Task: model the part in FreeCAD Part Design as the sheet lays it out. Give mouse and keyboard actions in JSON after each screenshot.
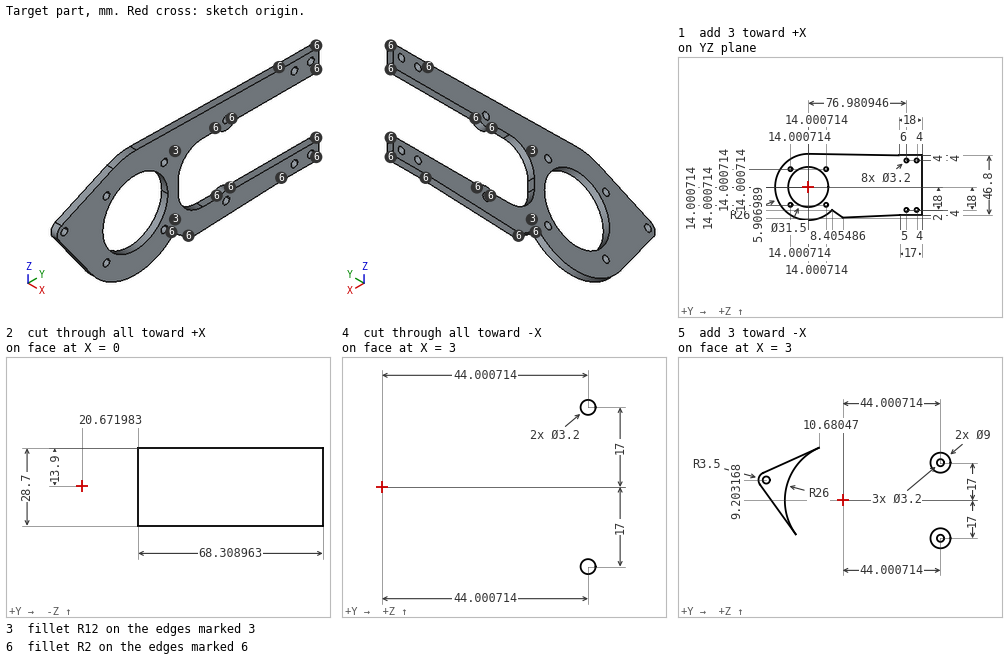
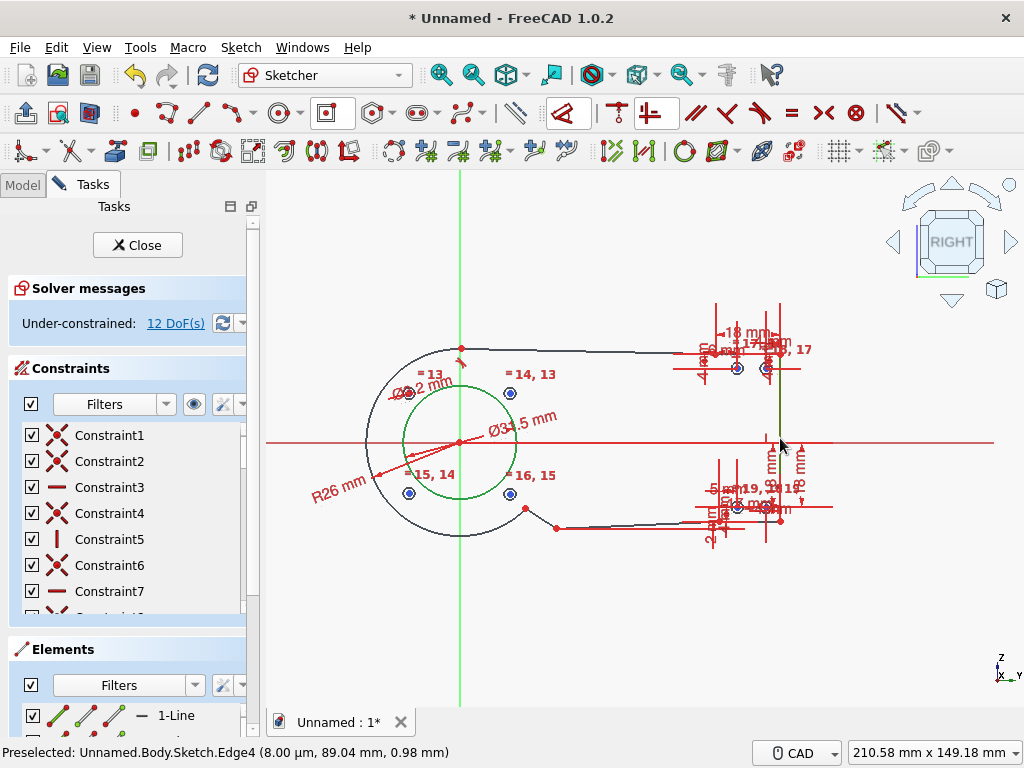
{"action": "left_click", "coordinate": [586, 114]}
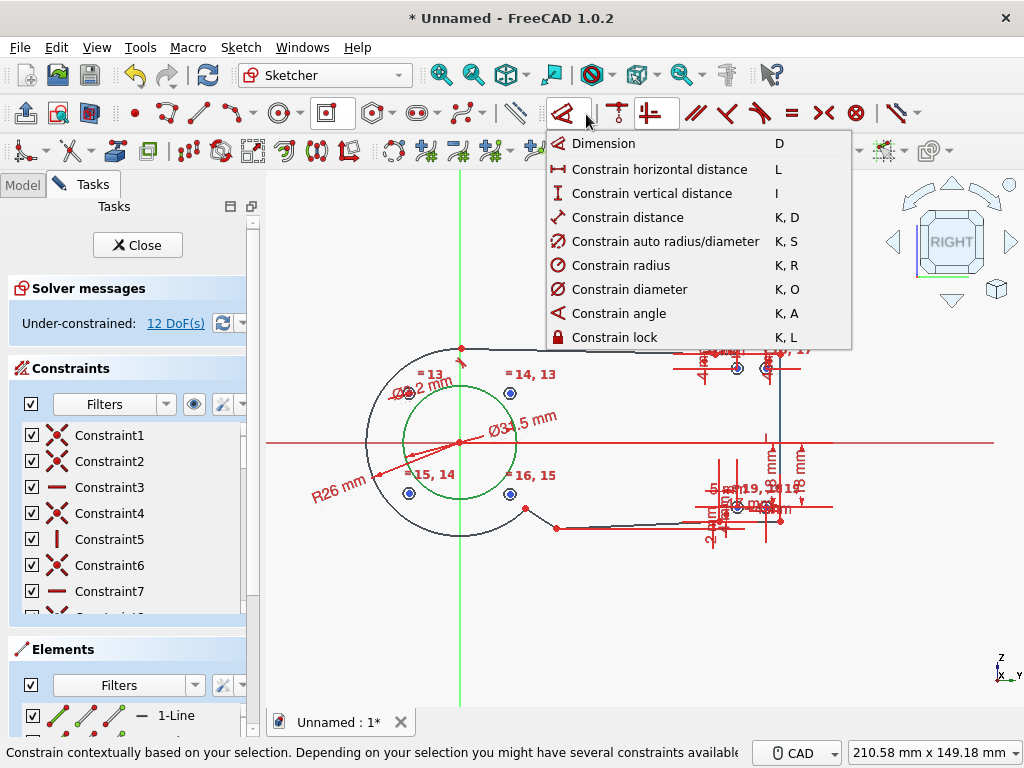
{"action": "left_click", "coordinate": [699, 193]}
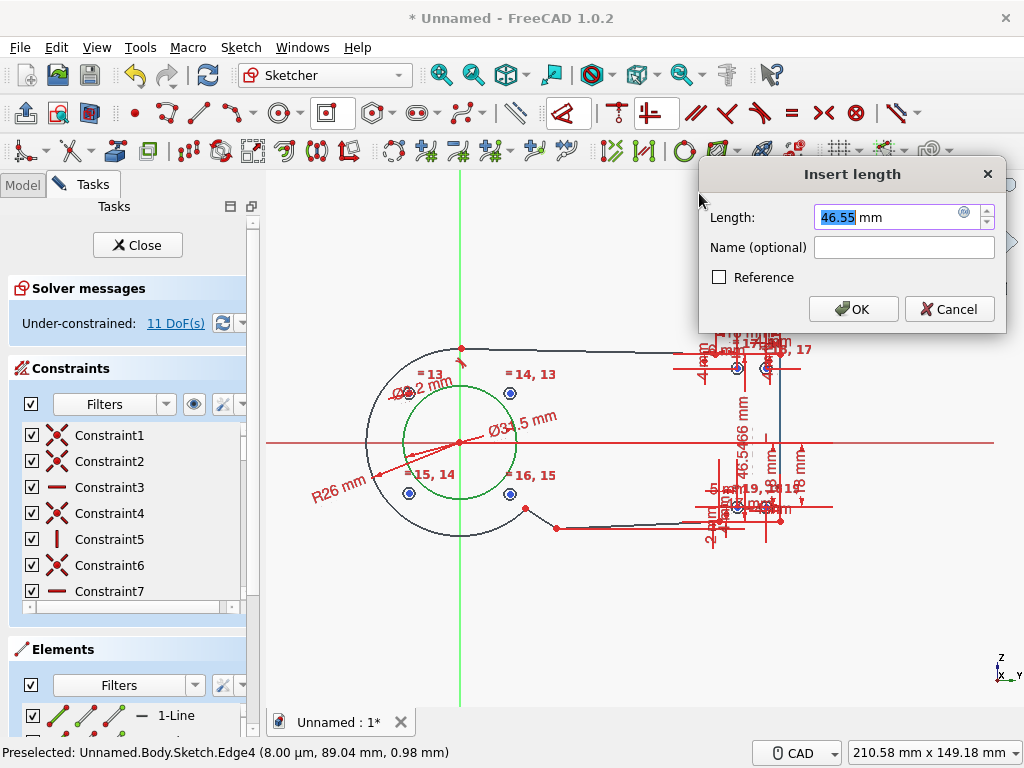
{"action": "type", "text": "46.8"}
{"action": "key", "text": "Return"}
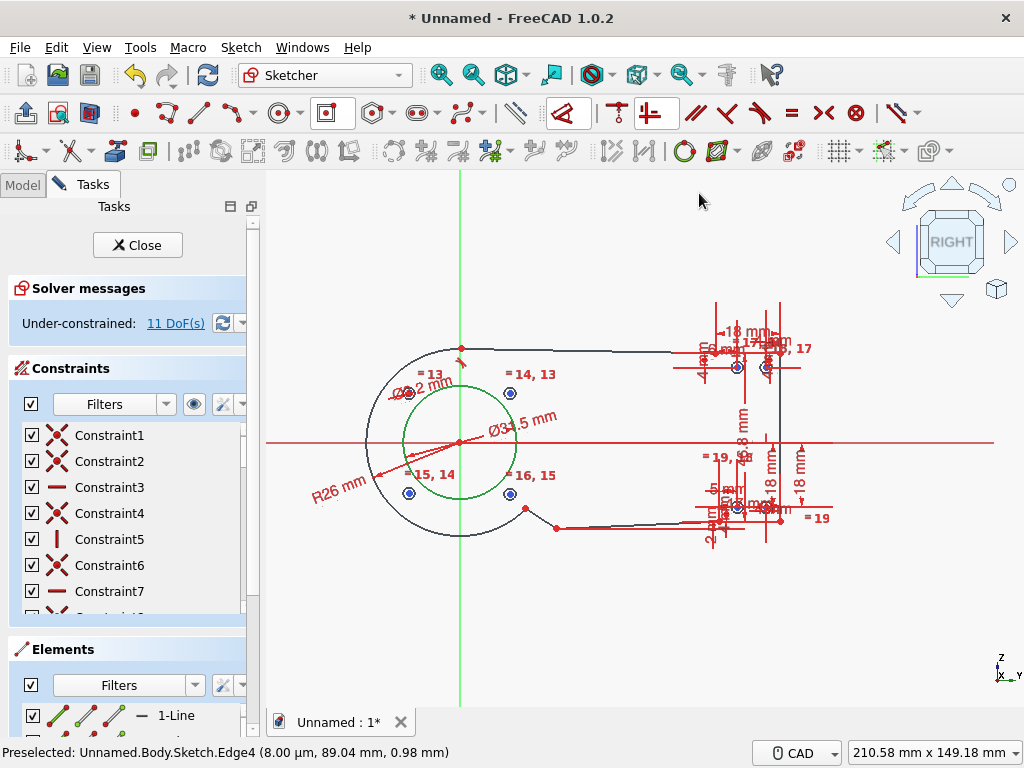
{"action": "scroll", "coordinate": [535, 515], "scroll_direction": "up", "scroll_amount": 2}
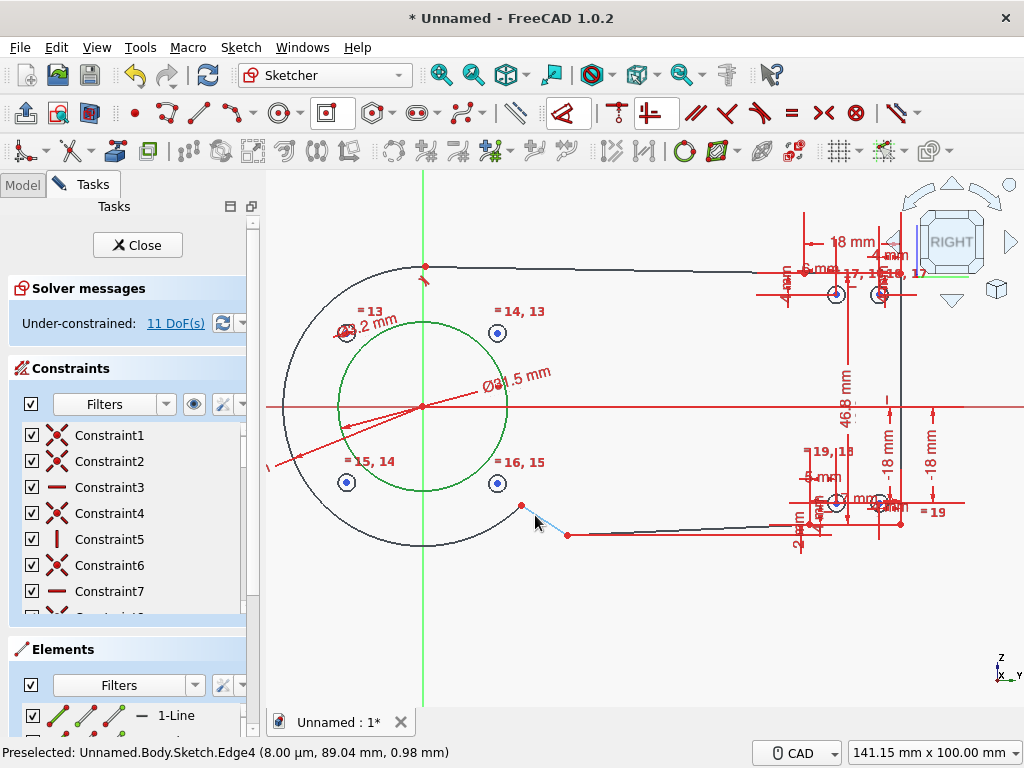
{"action": "left_click", "coordinate": [535, 514]}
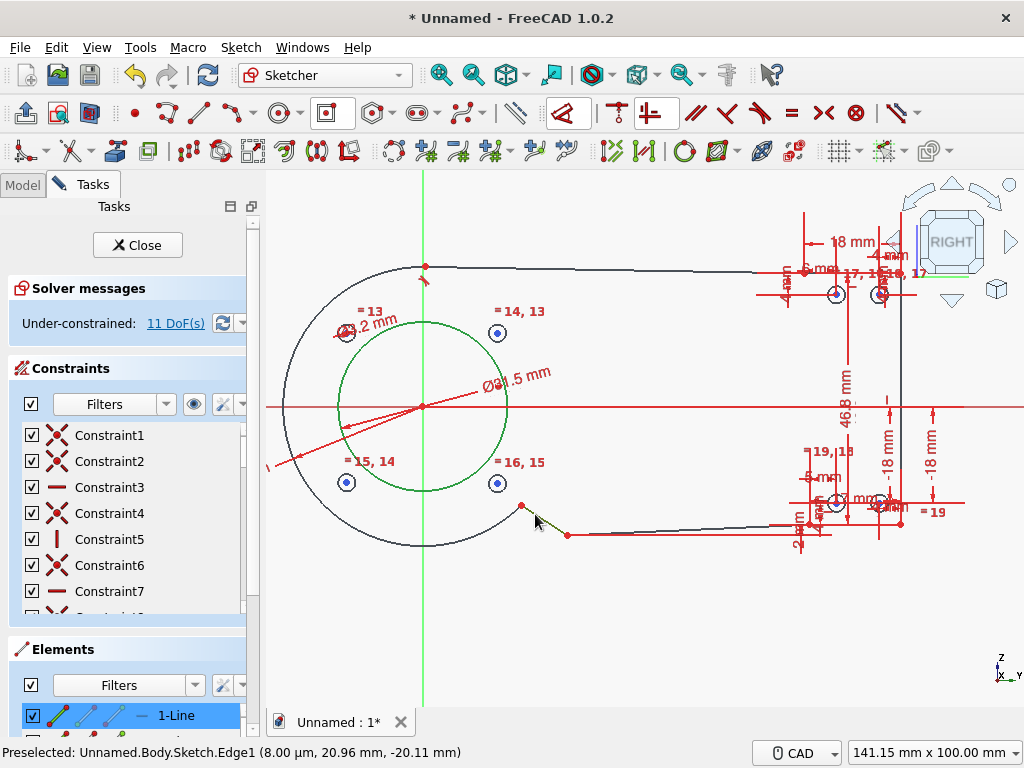
{"action": "left_click", "coordinate": [586, 114]}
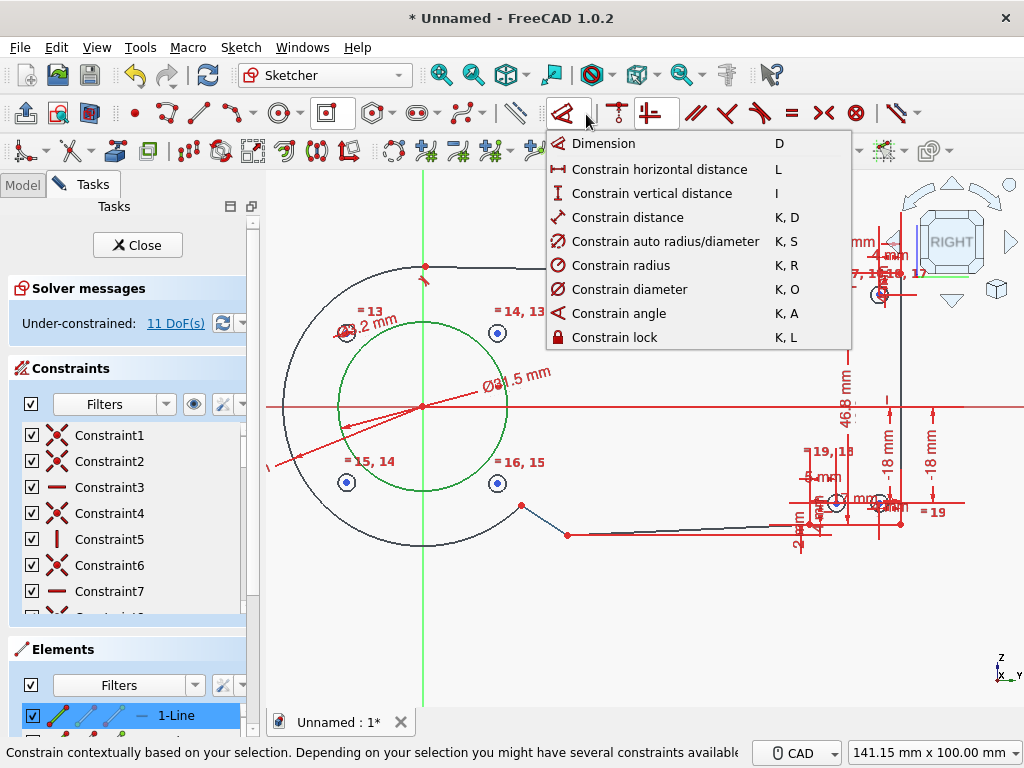
{"action": "left_click", "coordinate": [699, 169]}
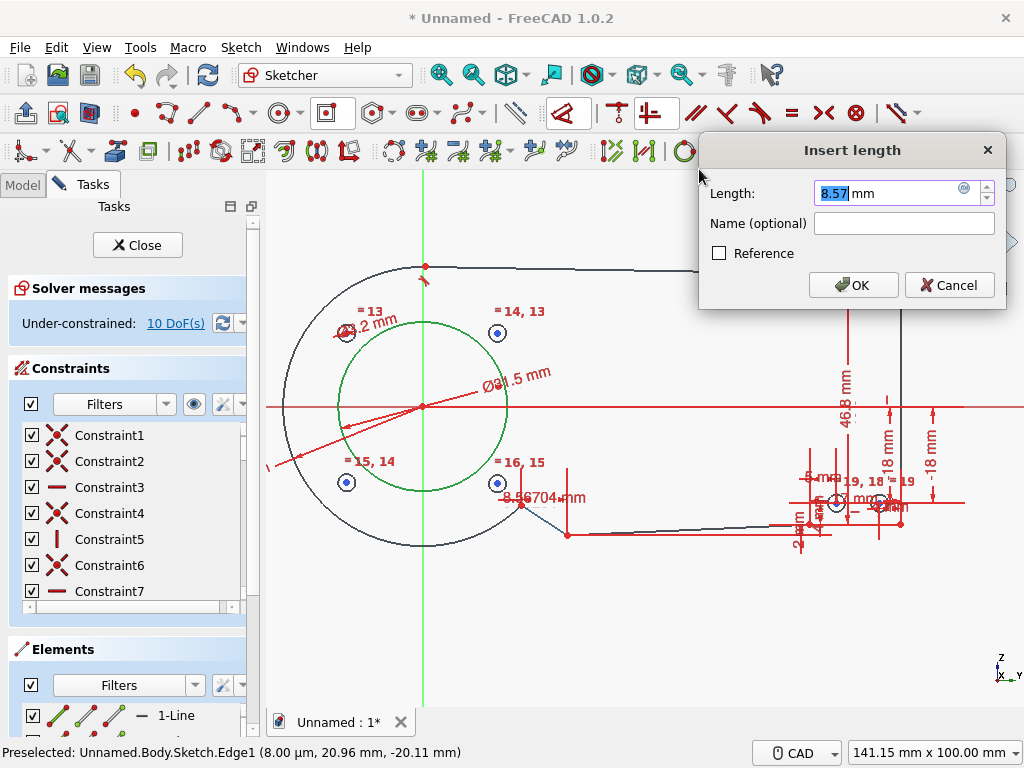
{"action": "type", "text": "8.405486"}
{"action": "key", "text": "Return"}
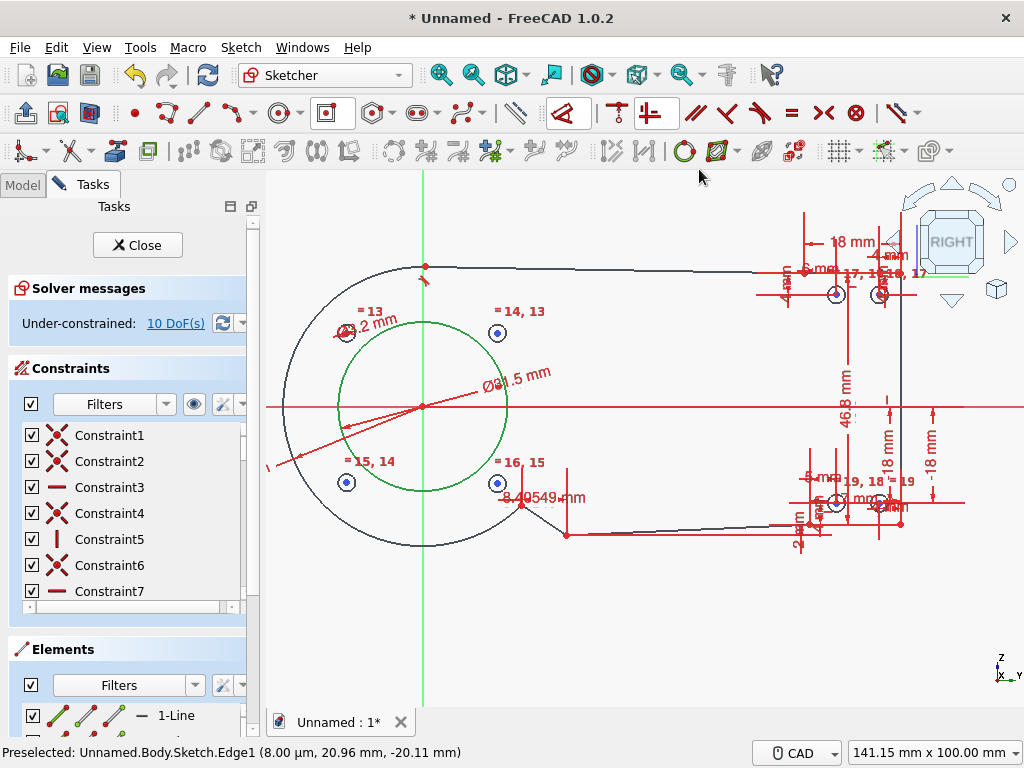
{"action": "scroll", "coordinate": [535, 514], "scroll_direction": "up", "scroll_amount": 2}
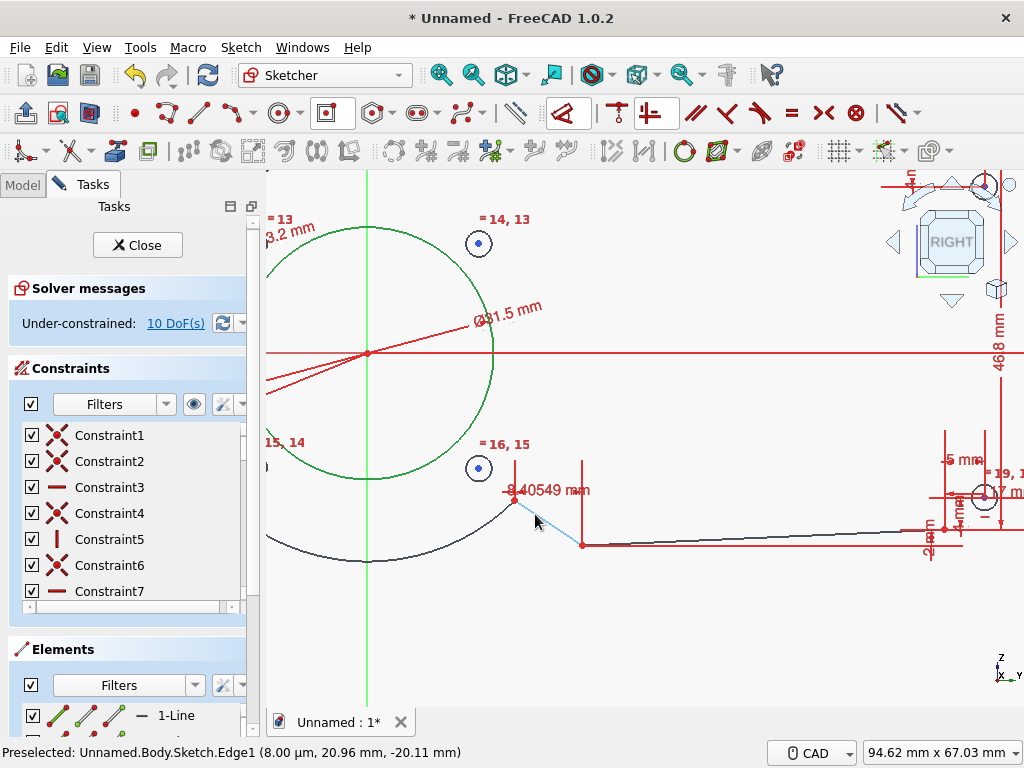
{"action": "left_click", "coordinate": [535, 514]}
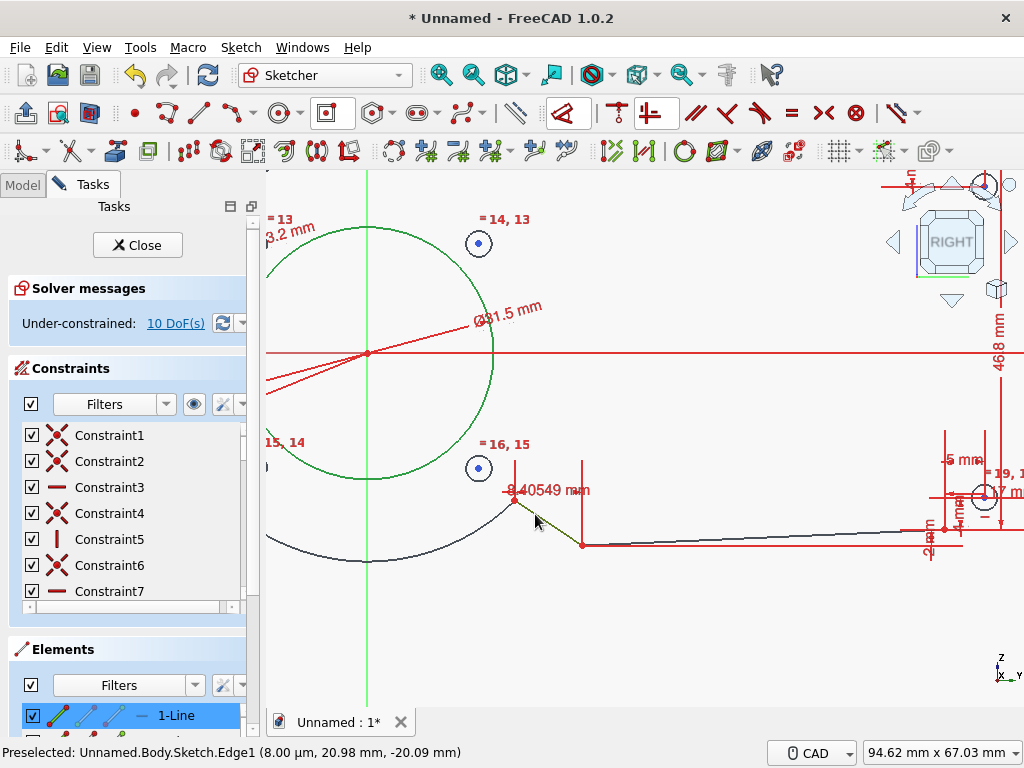
{"action": "left_click", "coordinate": [586, 114]}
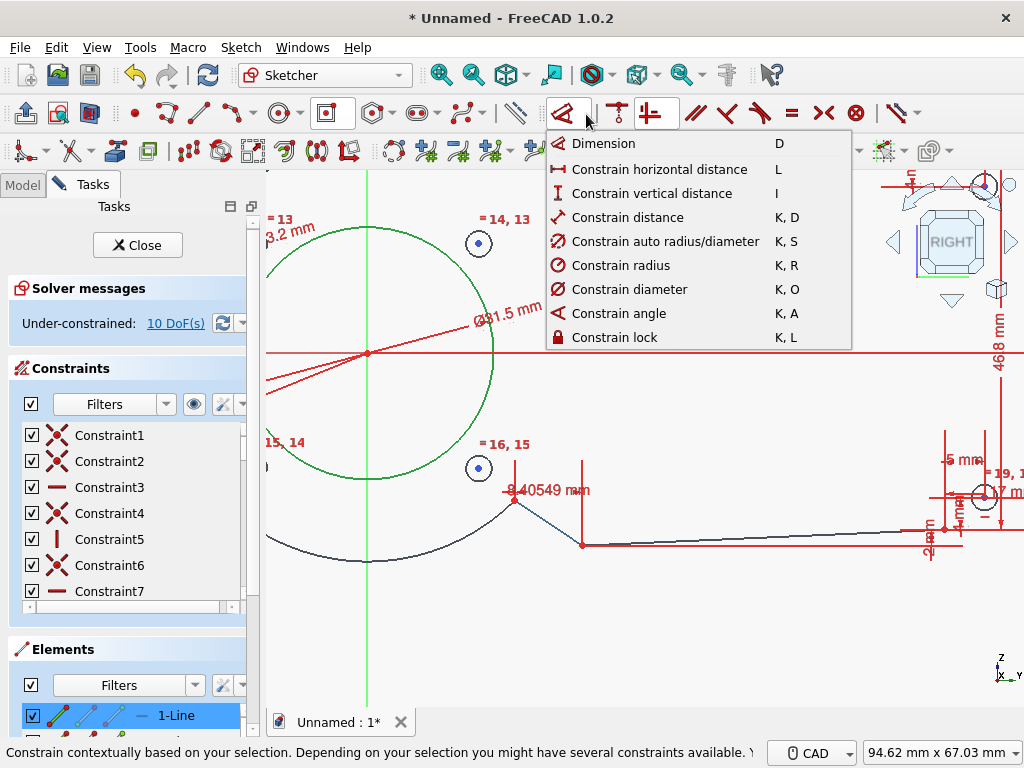
{"action": "left_click", "coordinate": [699, 193]}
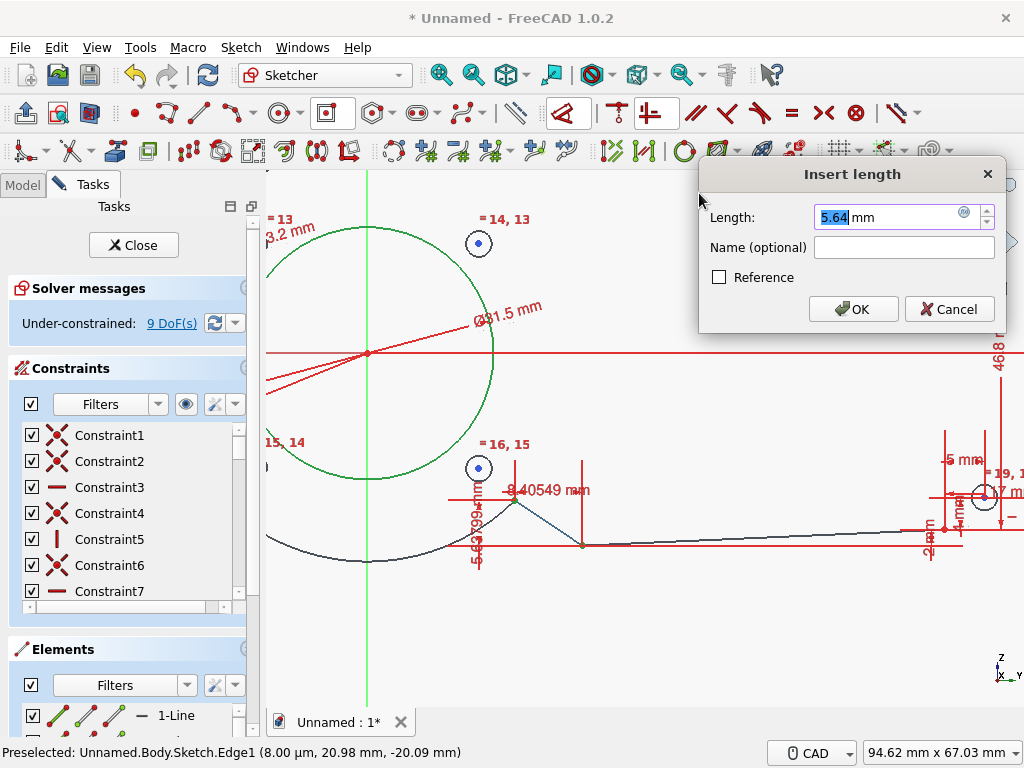
{"action": "type", "text": "5.906989"}
{"action": "key", "text": "Return"}